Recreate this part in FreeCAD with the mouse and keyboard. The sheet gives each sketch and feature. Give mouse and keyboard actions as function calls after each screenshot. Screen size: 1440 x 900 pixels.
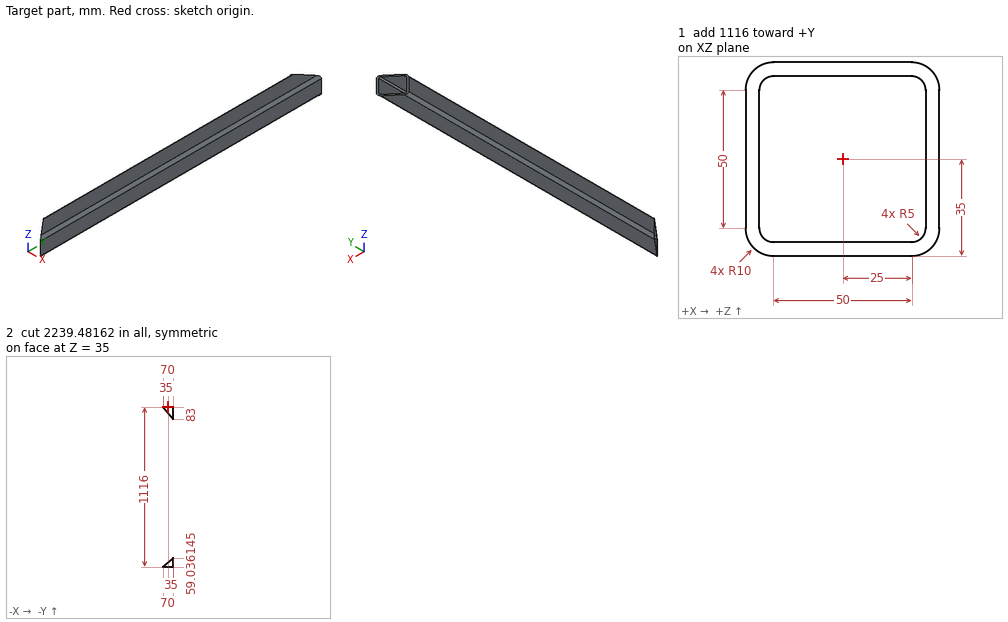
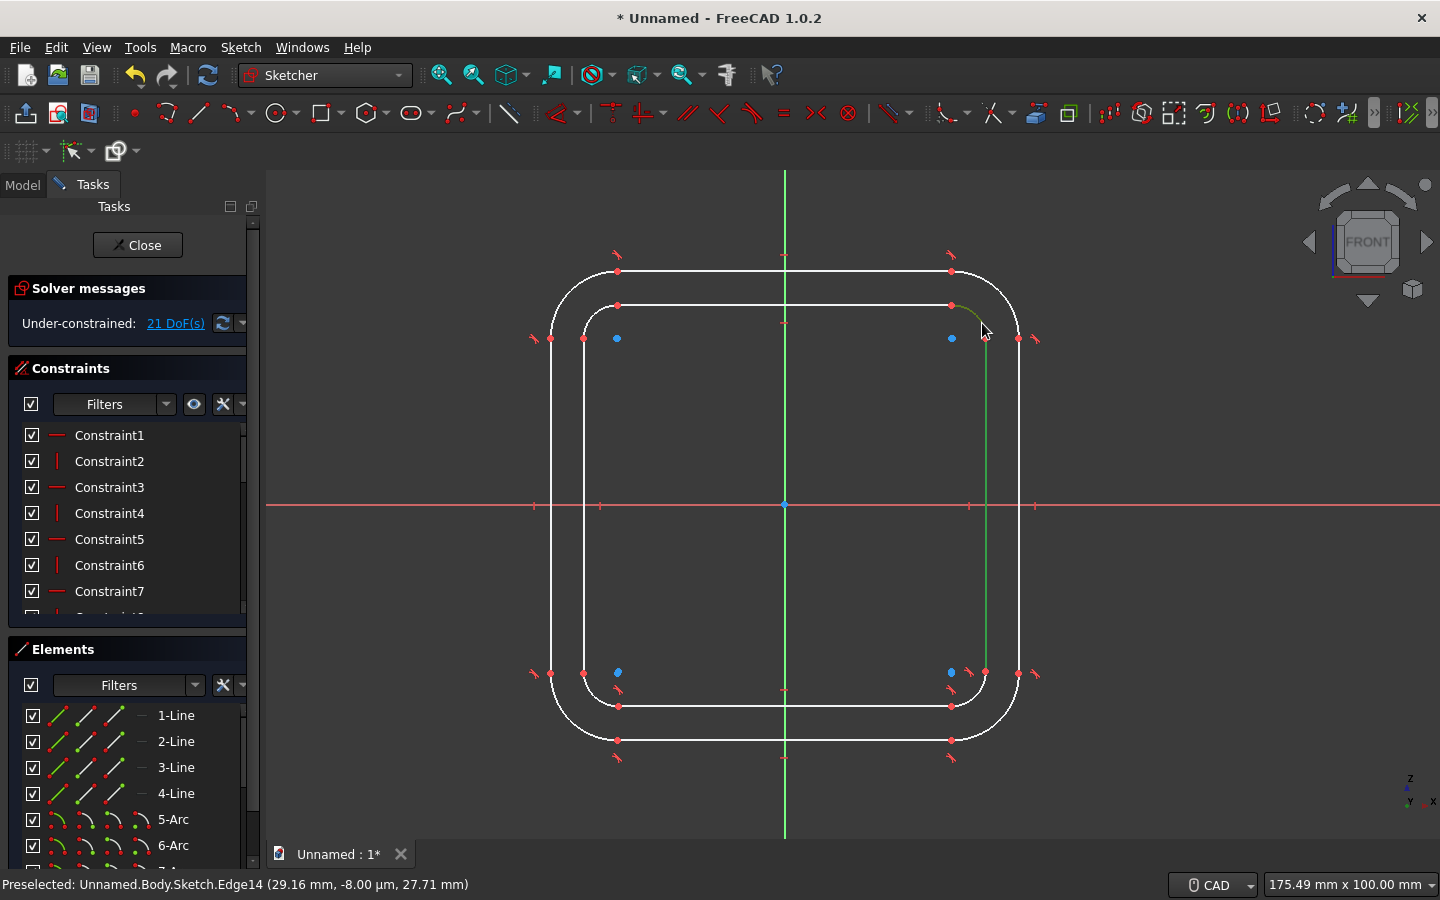
key(t)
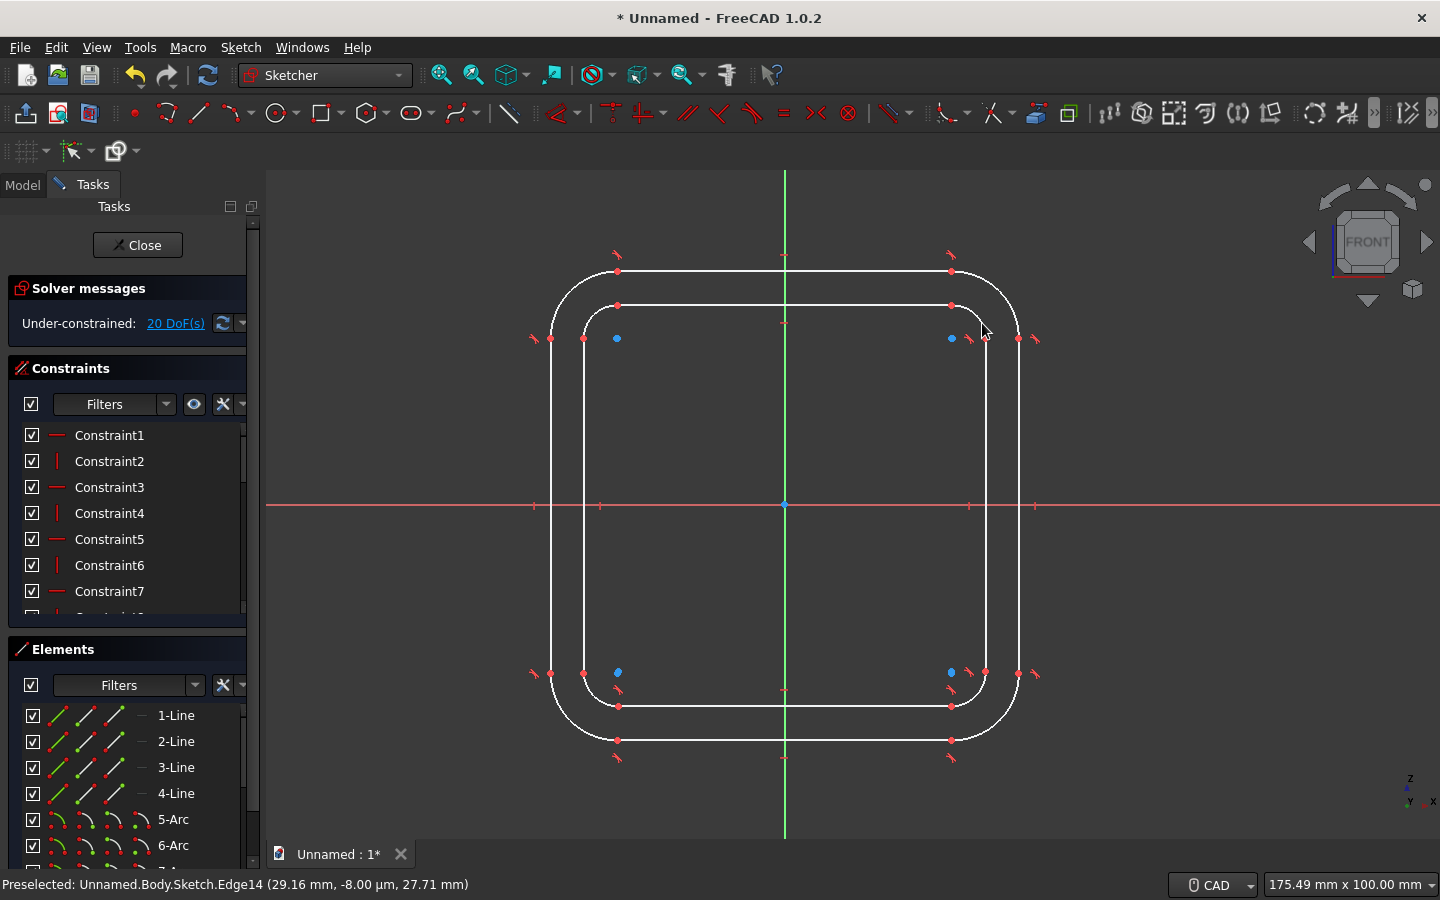
click(852, 305)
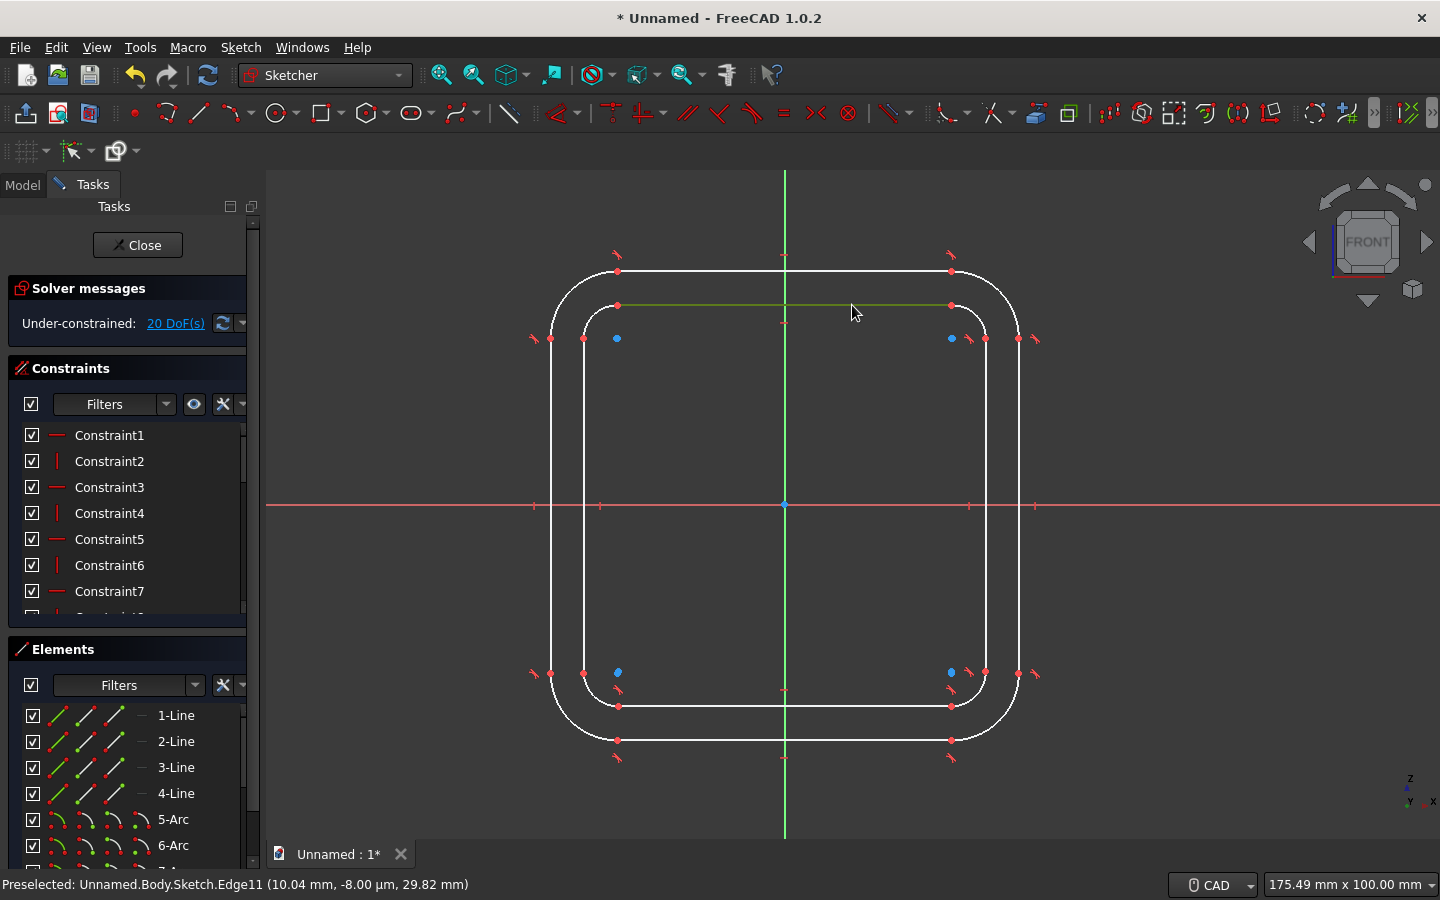
click(982, 323)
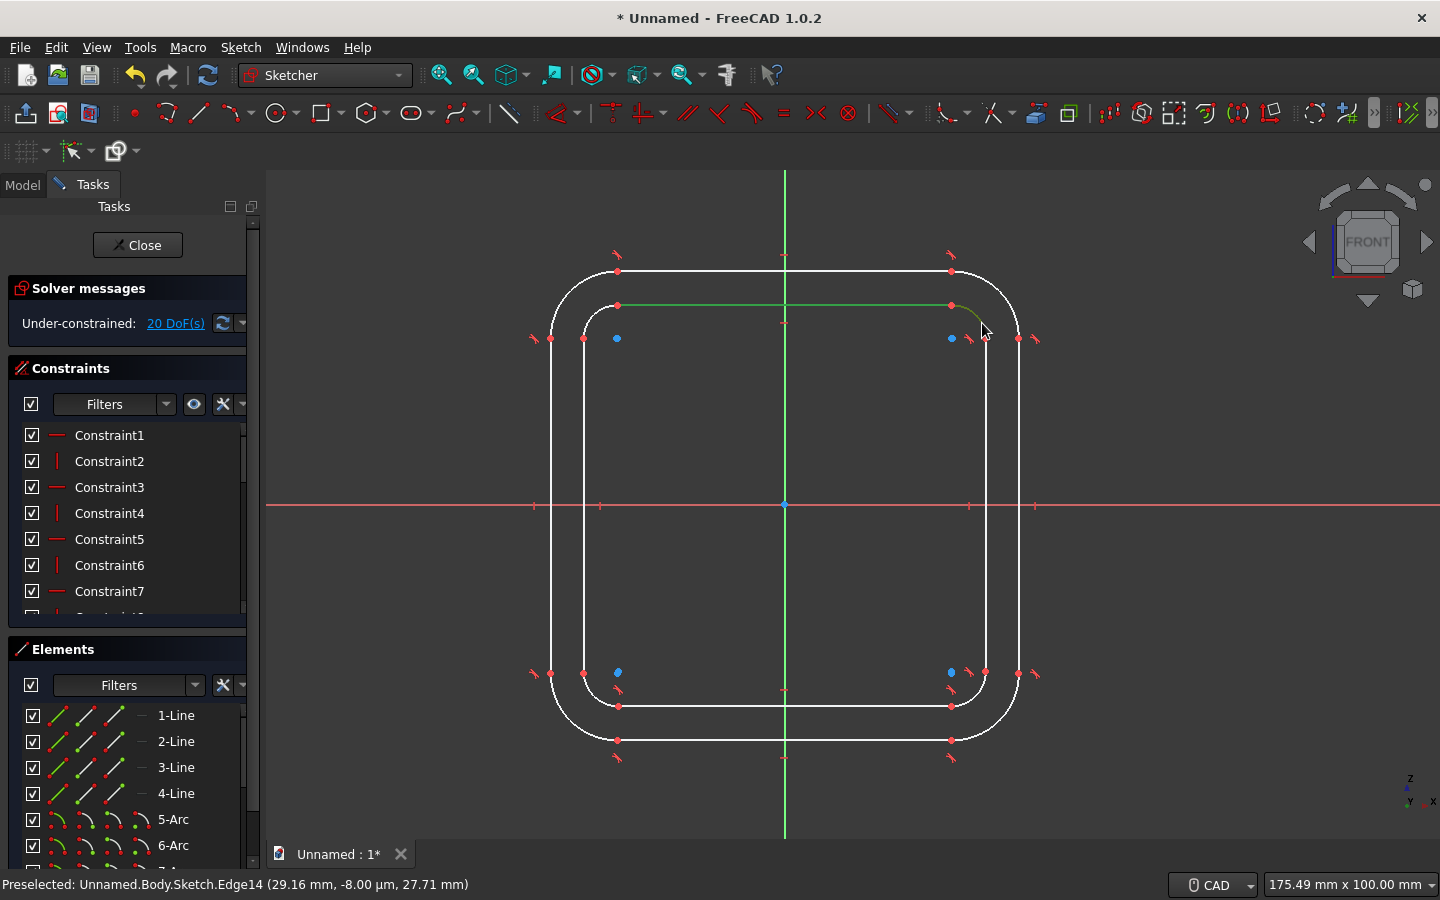
key(t)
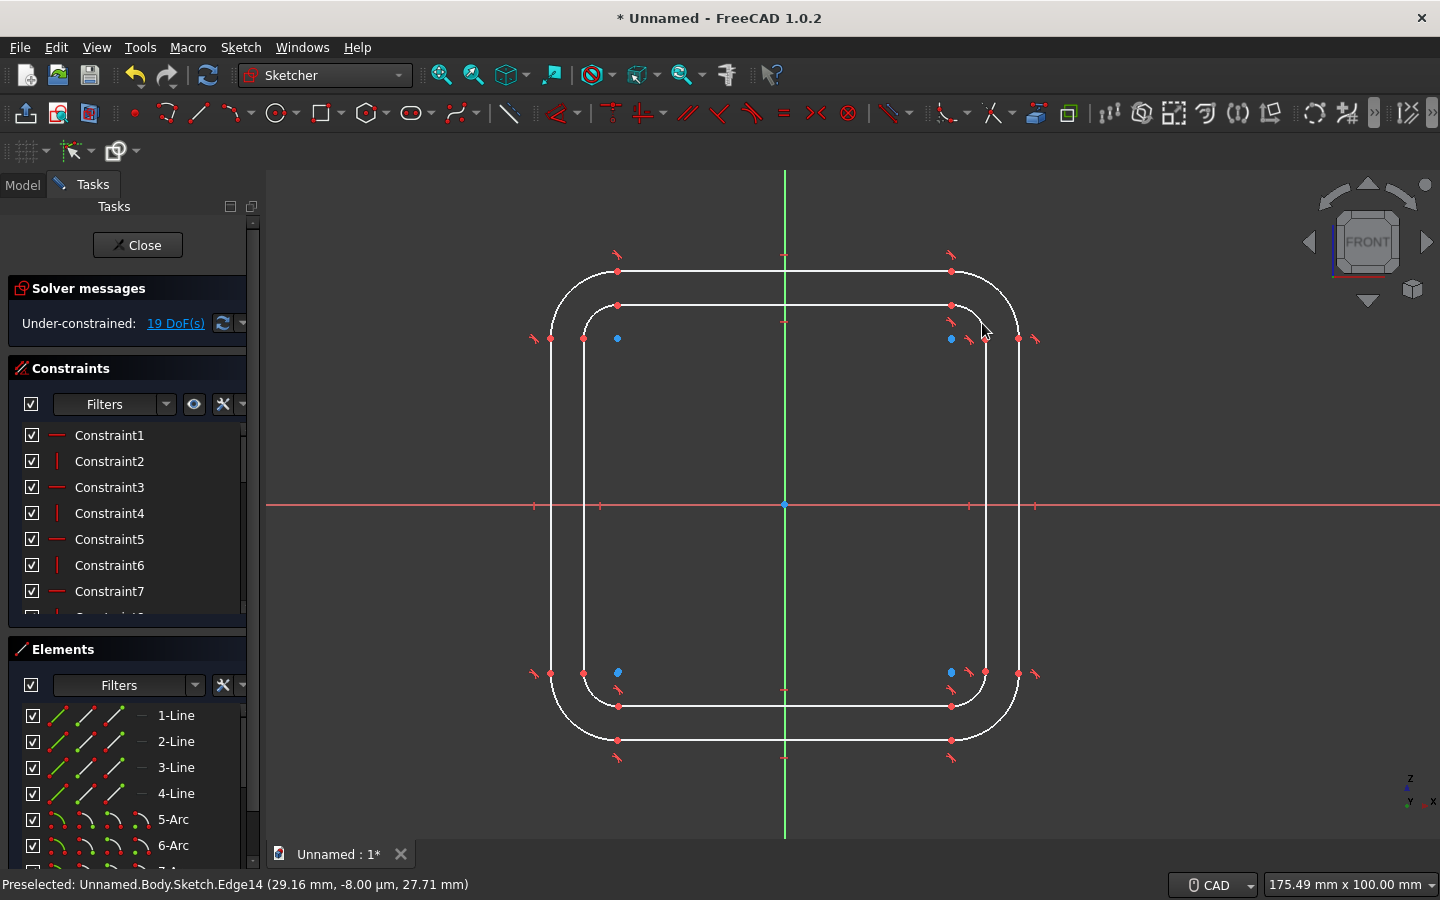
click(852, 305)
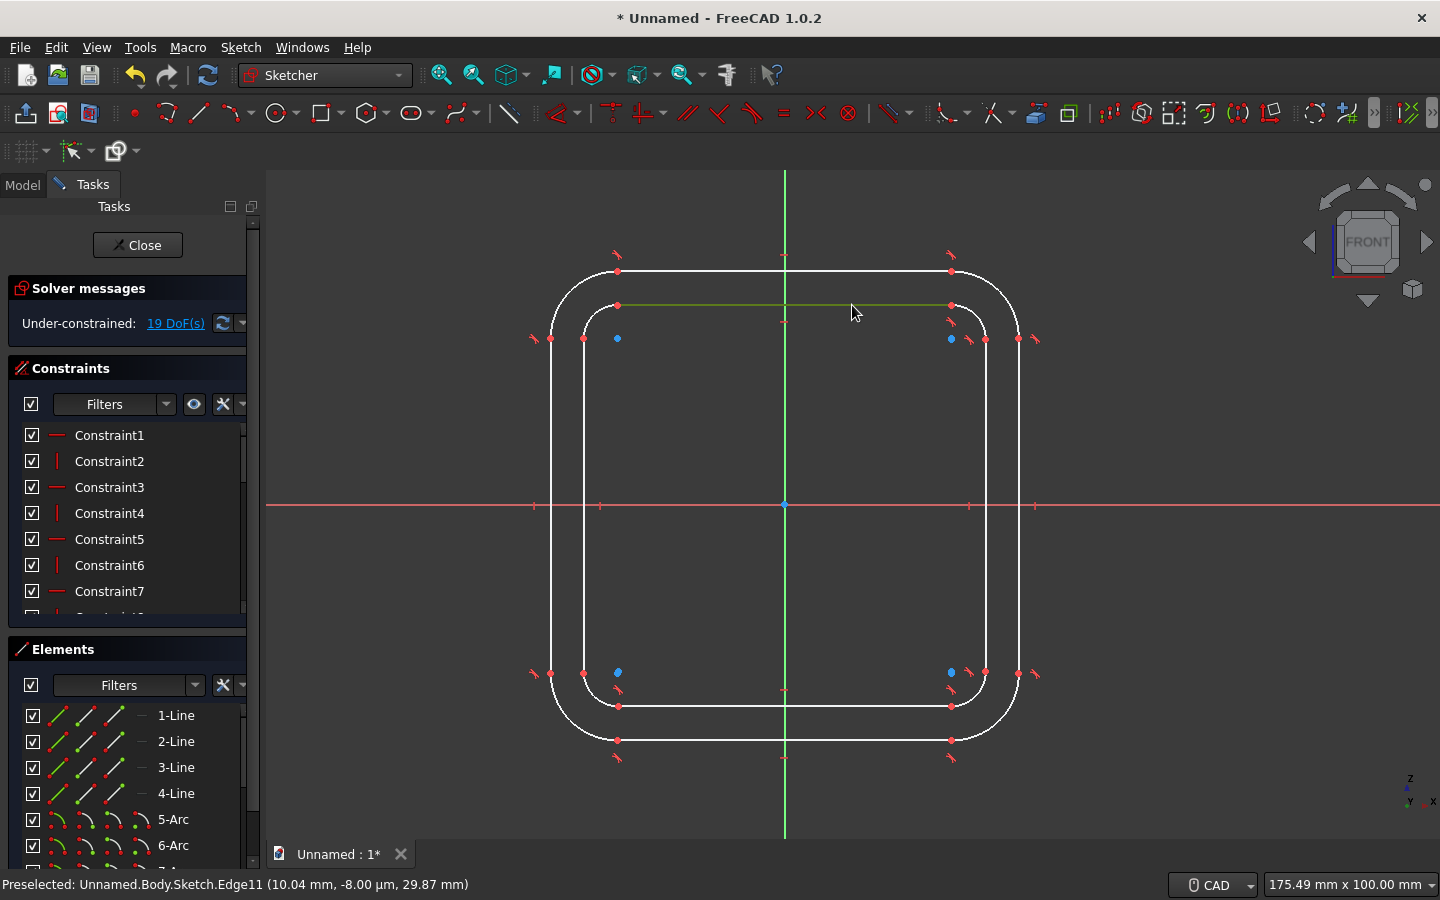
click(602, 309)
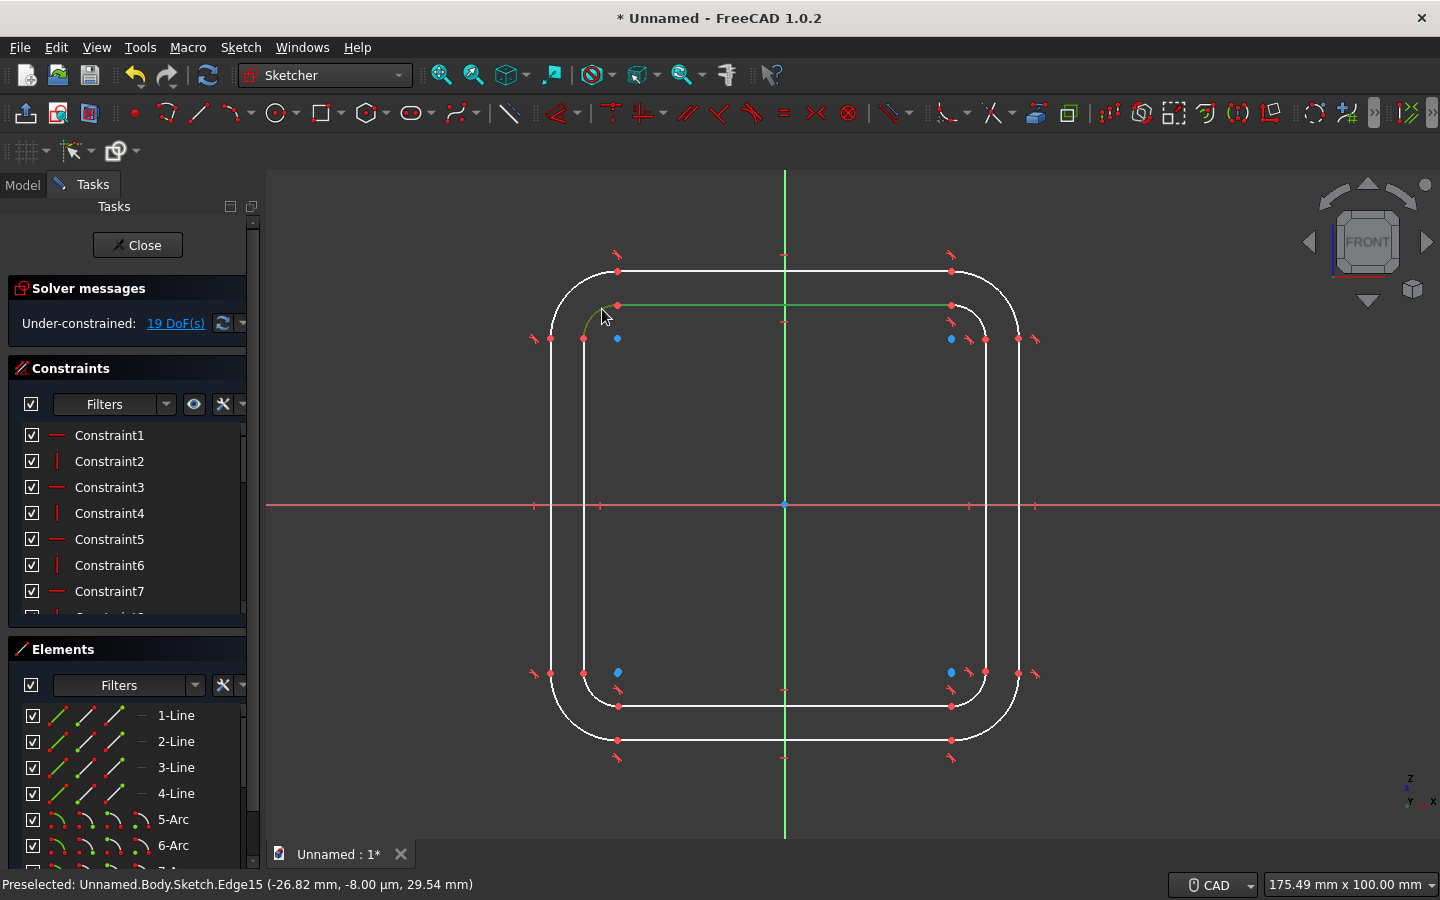
key(t)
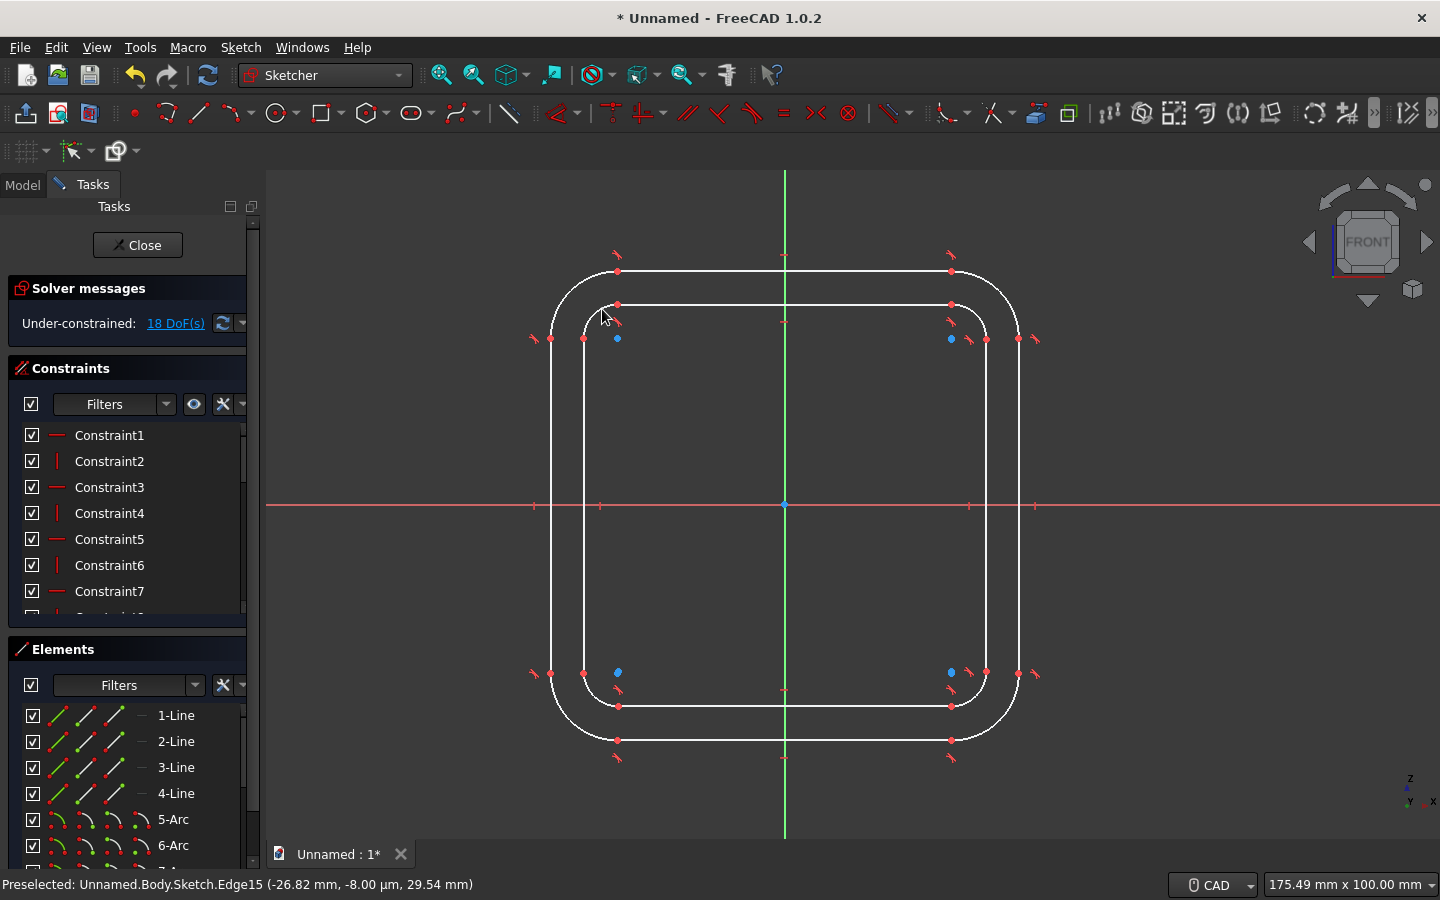
click(584, 439)